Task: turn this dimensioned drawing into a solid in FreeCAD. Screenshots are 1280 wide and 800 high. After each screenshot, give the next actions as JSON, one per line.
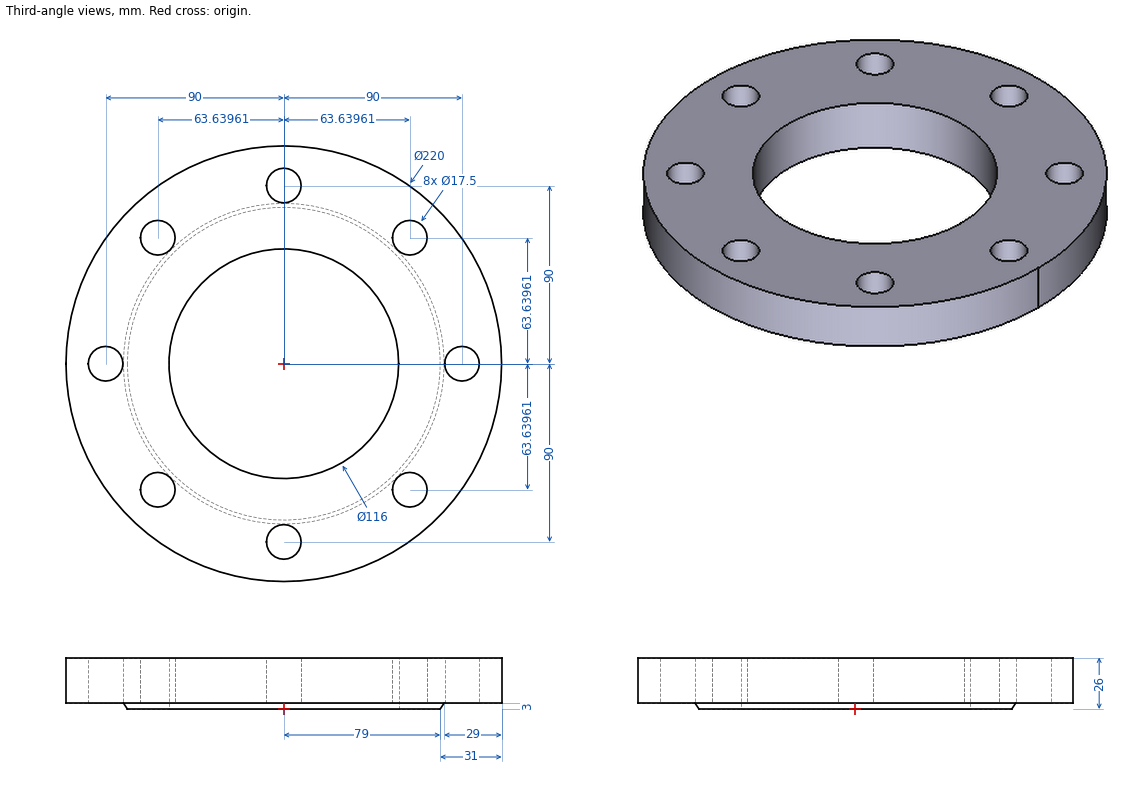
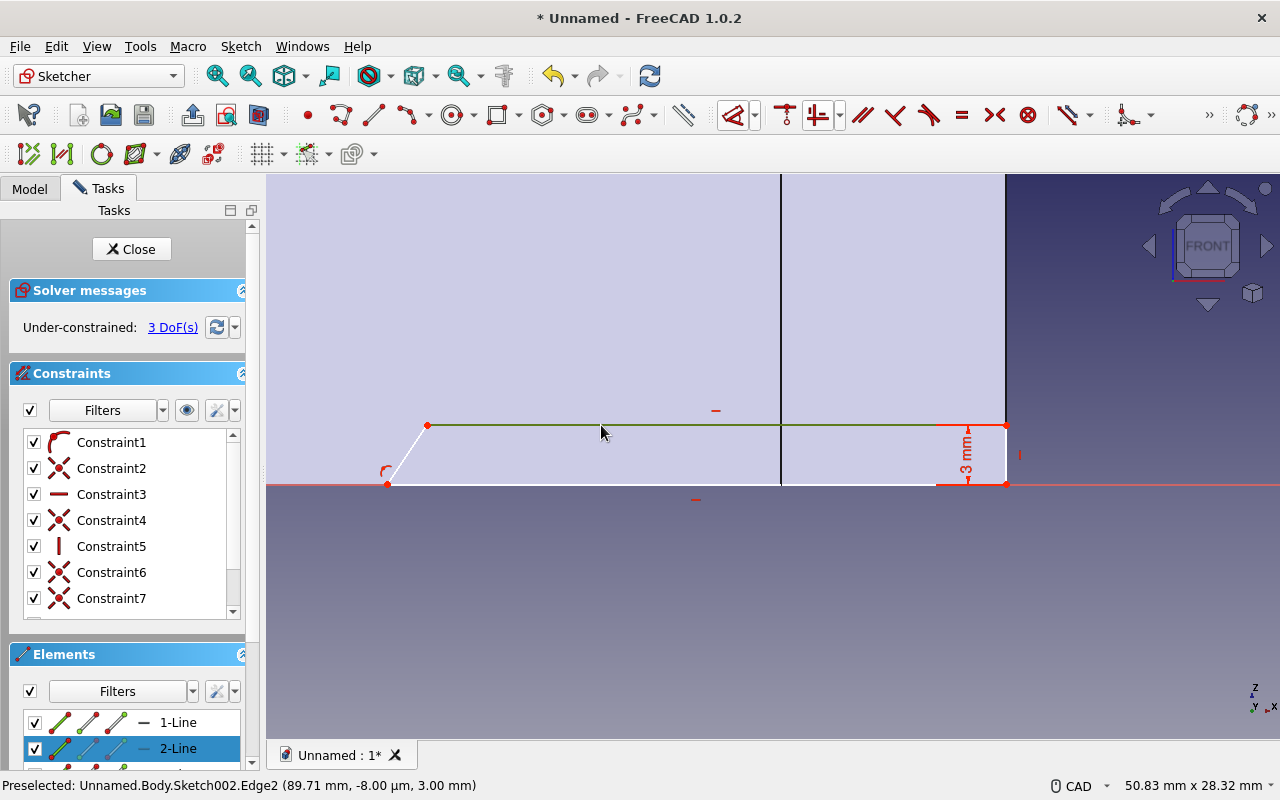
{"action": "key", "text": "l"}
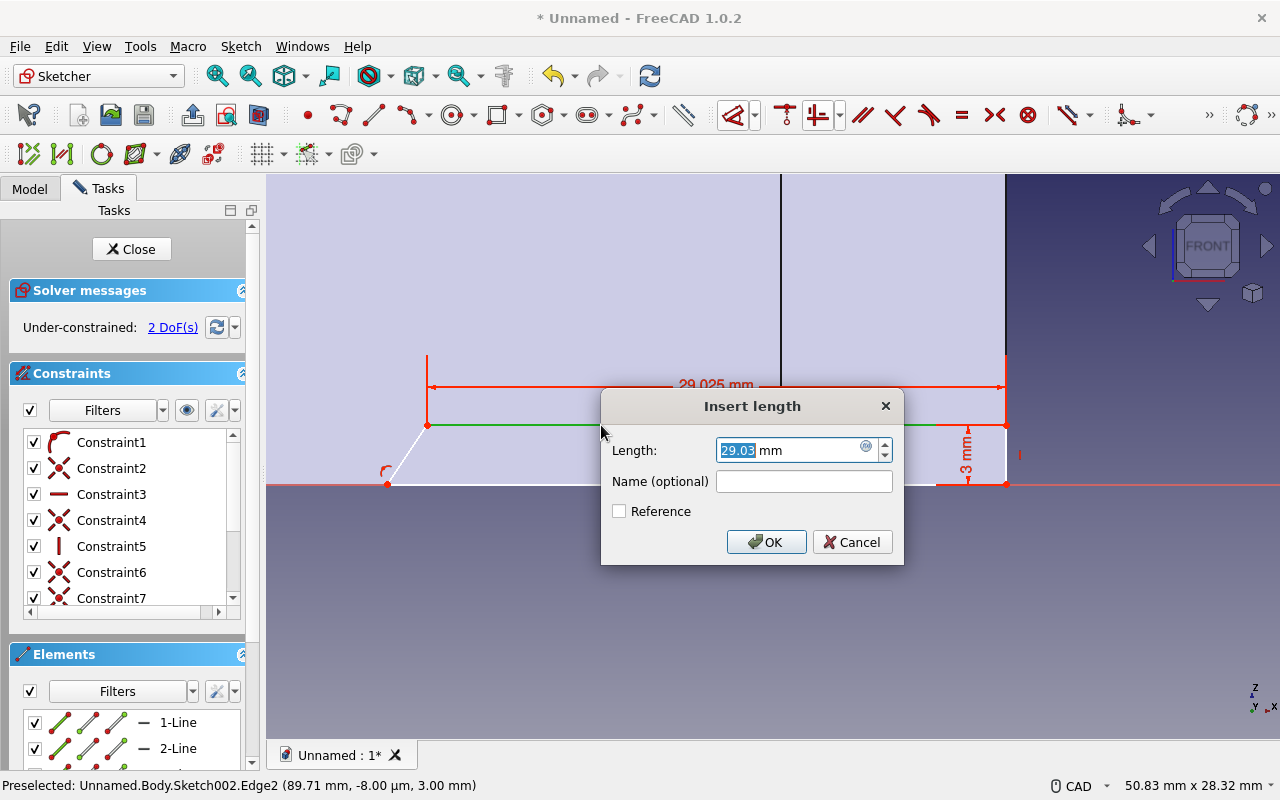
{"action": "type", "text": "29"}
{"action": "key", "text": "Return"}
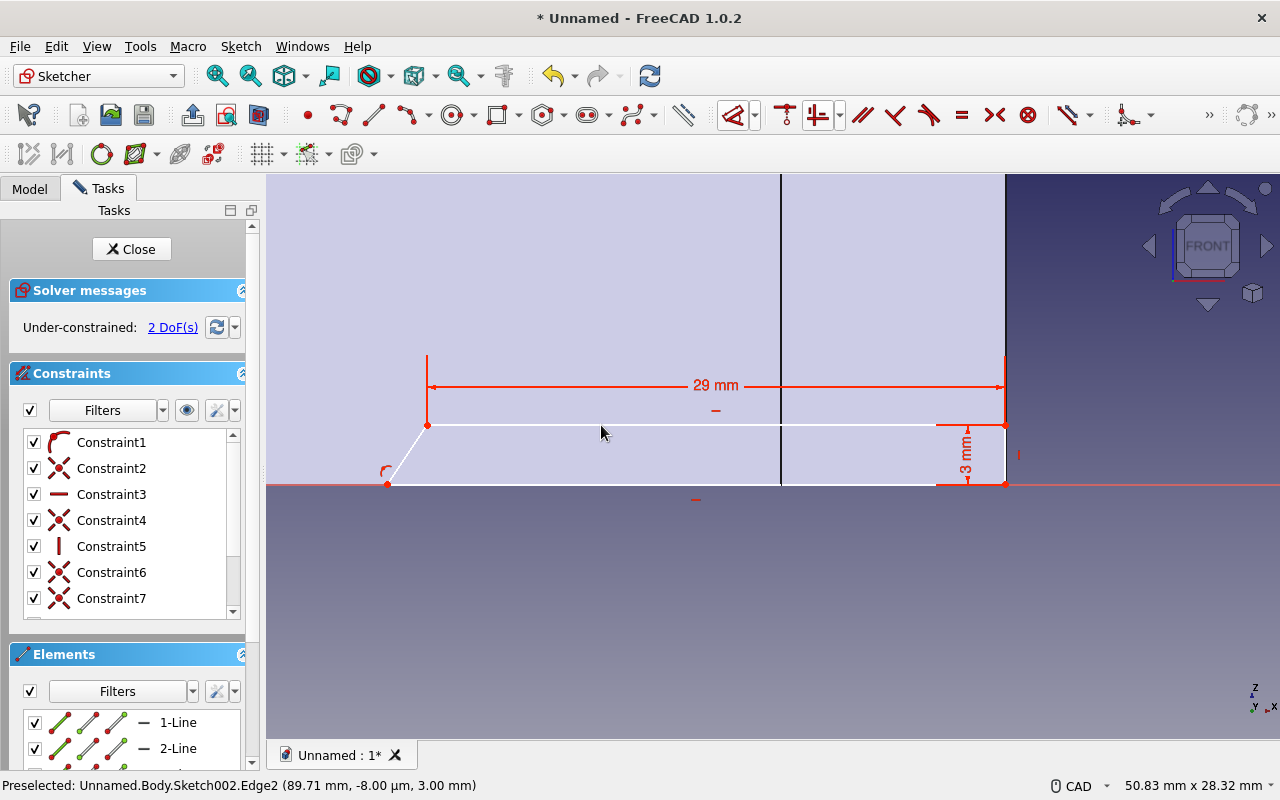
{"action": "left_click", "coordinate": [820, 485]}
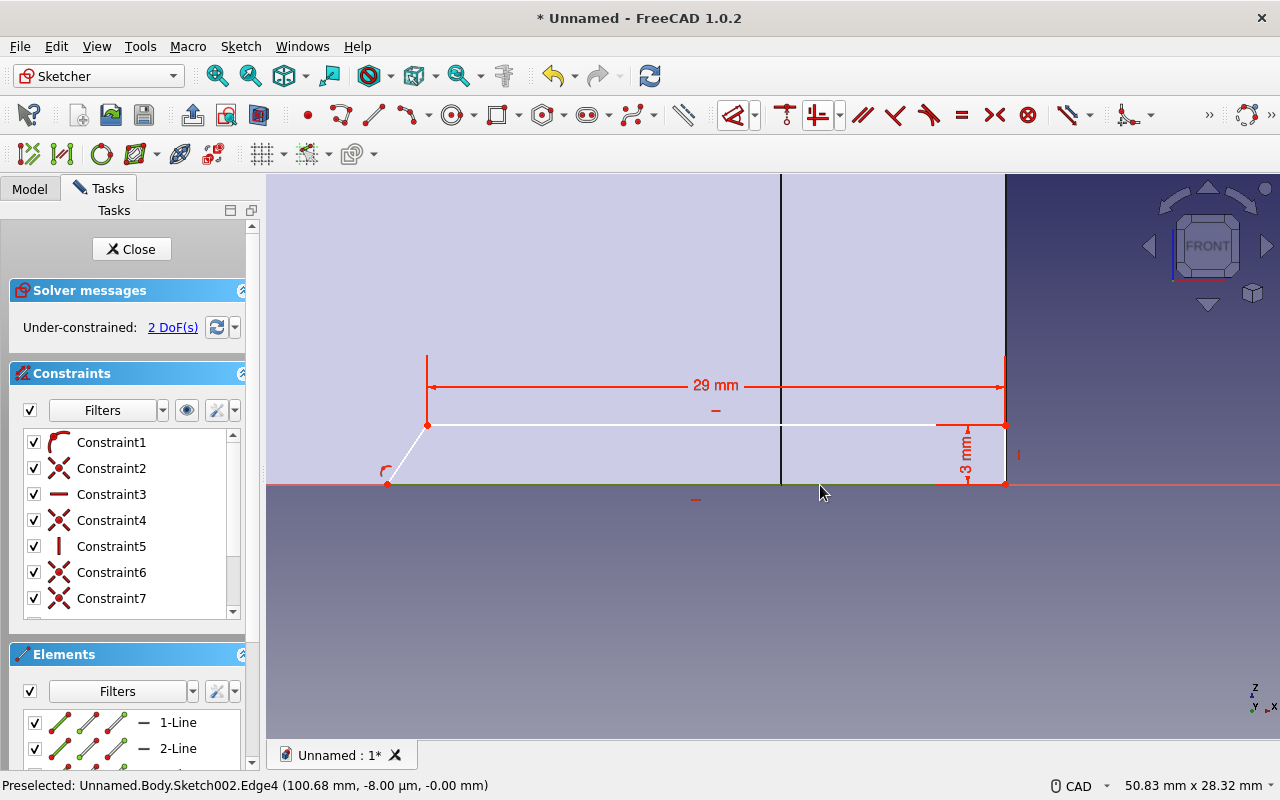
{"action": "key", "text": "l"}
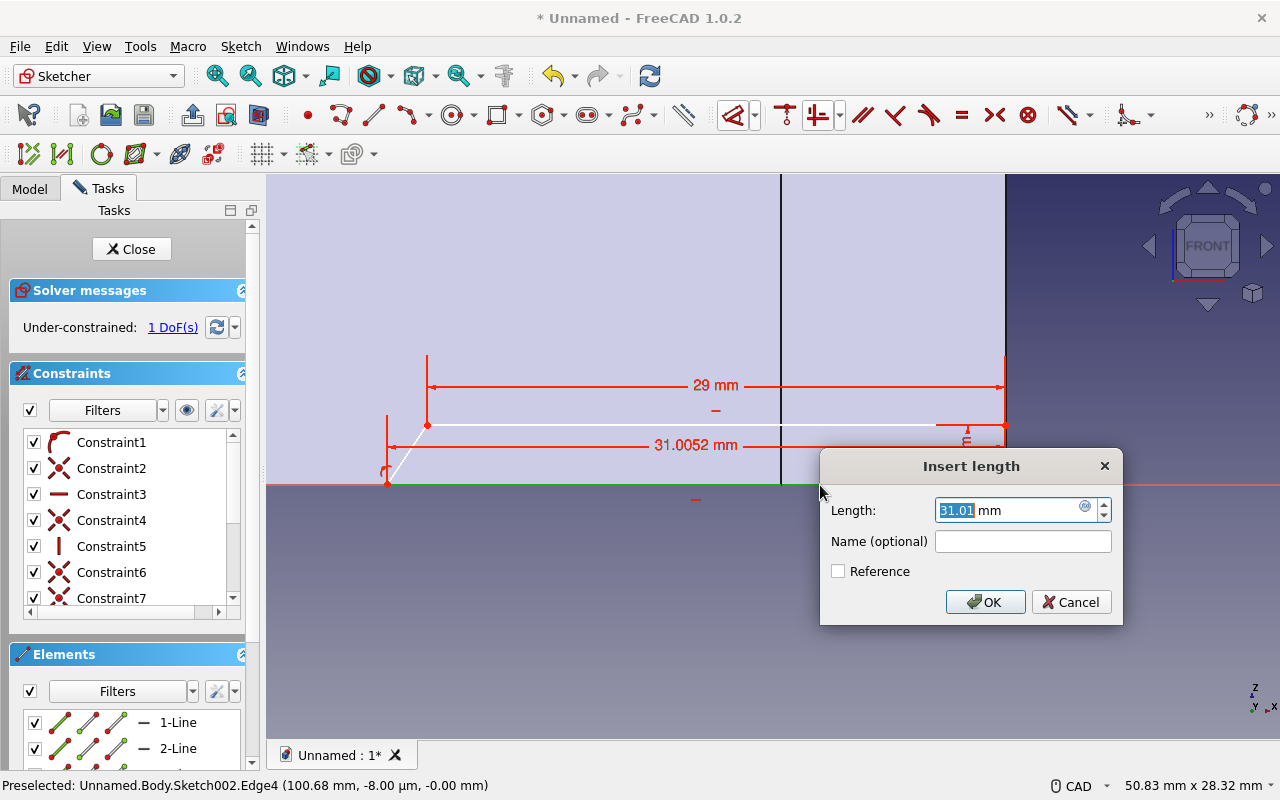
{"action": "type", "text": "31"}
{"action": "key", "text": "Return"}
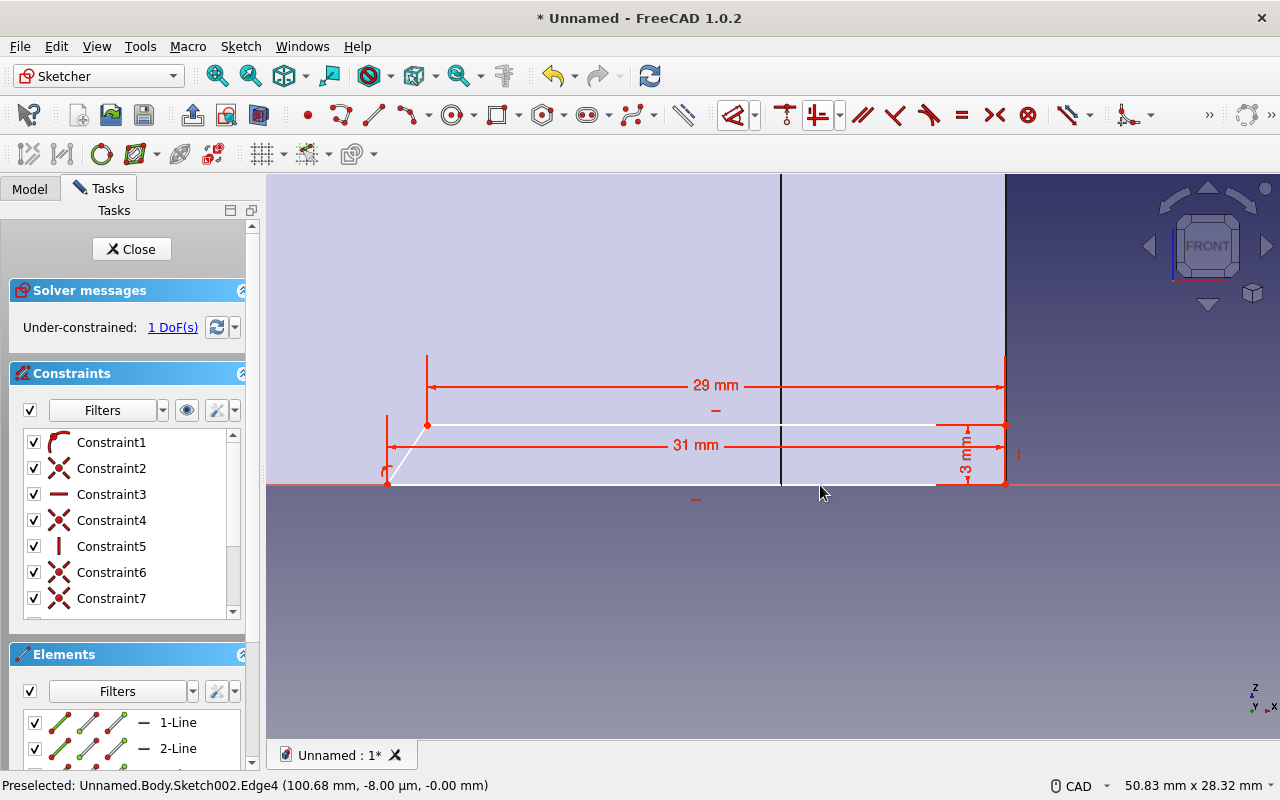
{"action": "left_click", "coordinate": [387, 485]}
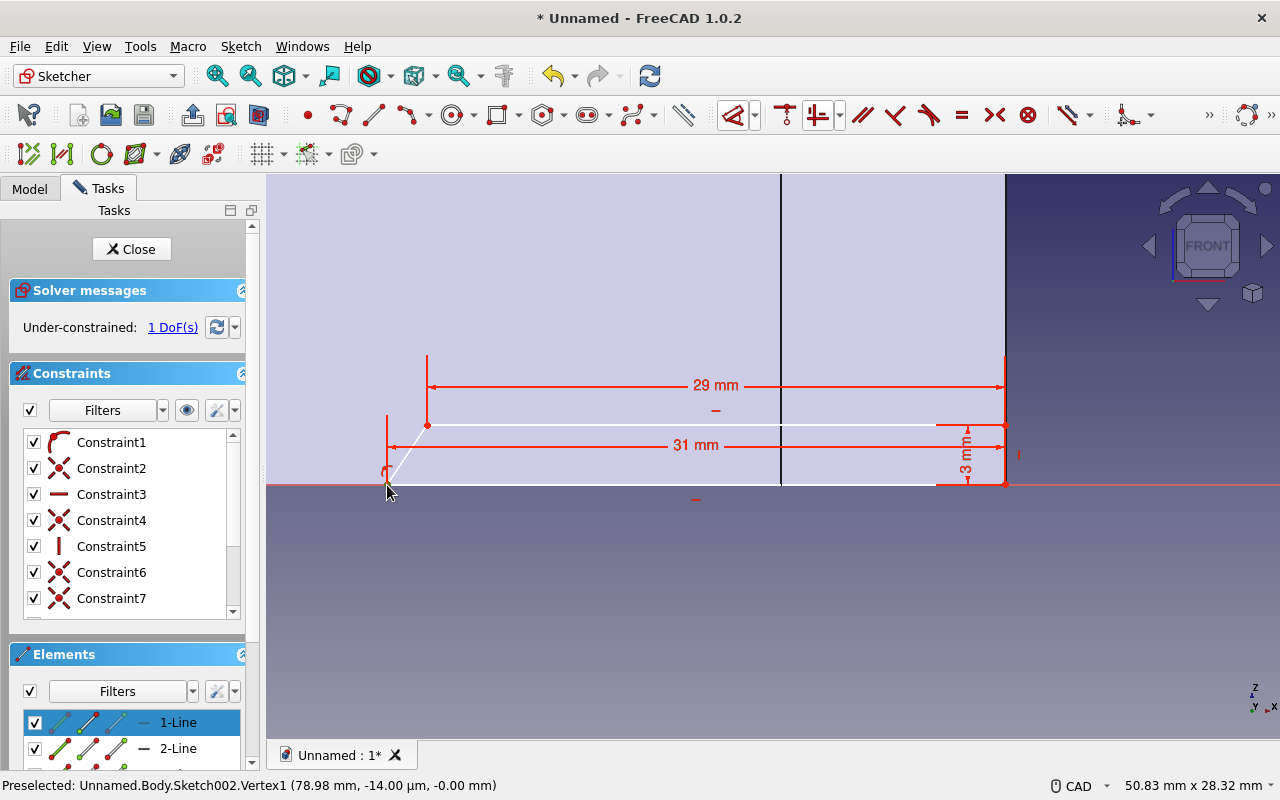
{"action": "left_click", "coordinate": [754, 116]}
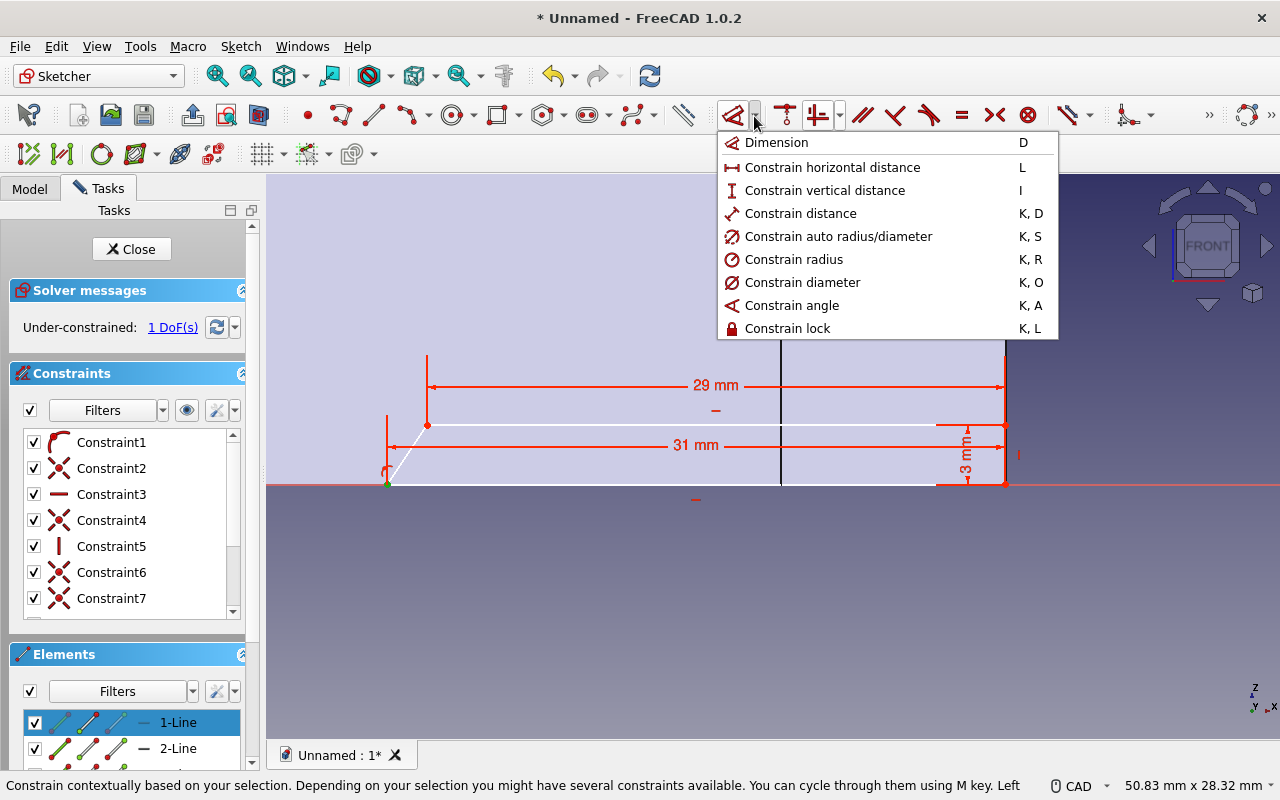
{"action": "left_click", "coordinate": [888, 168]}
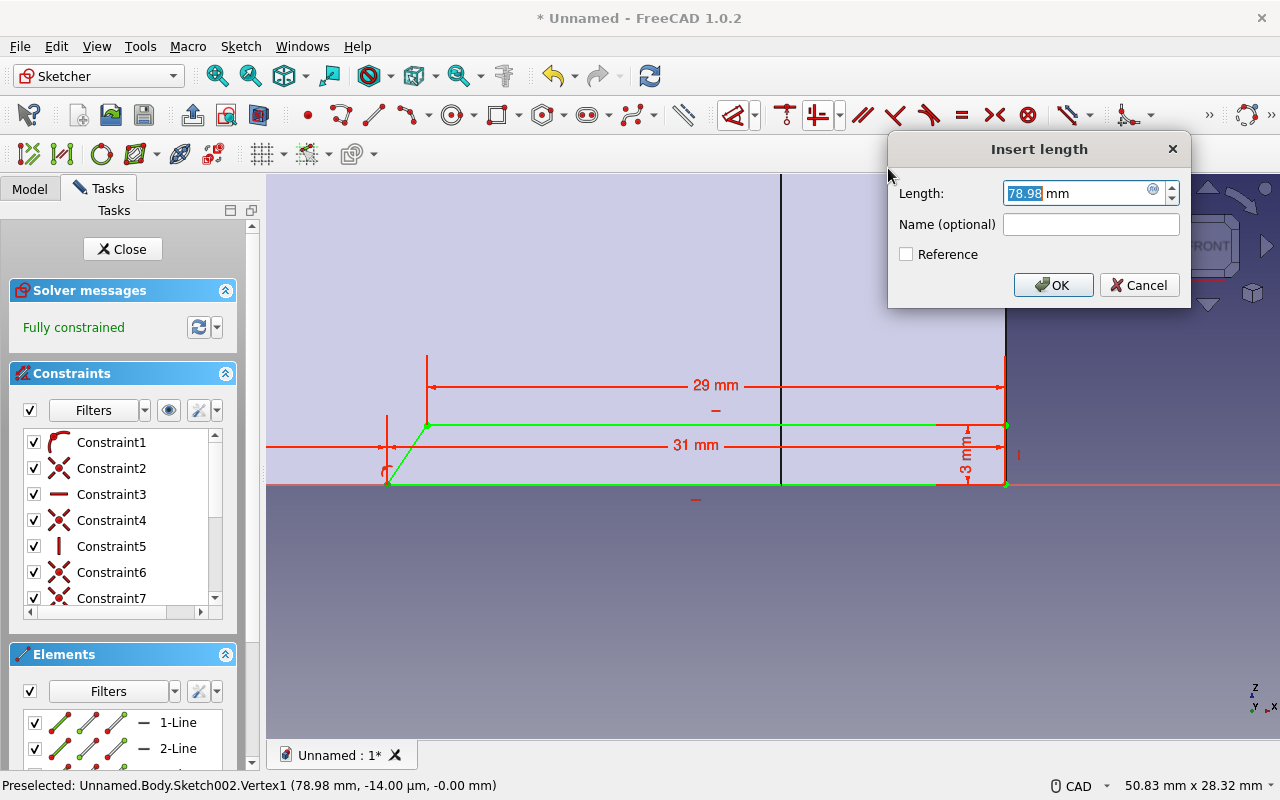
{"action": "type", "text": "79"}
{"action": "key", "text": "Return"}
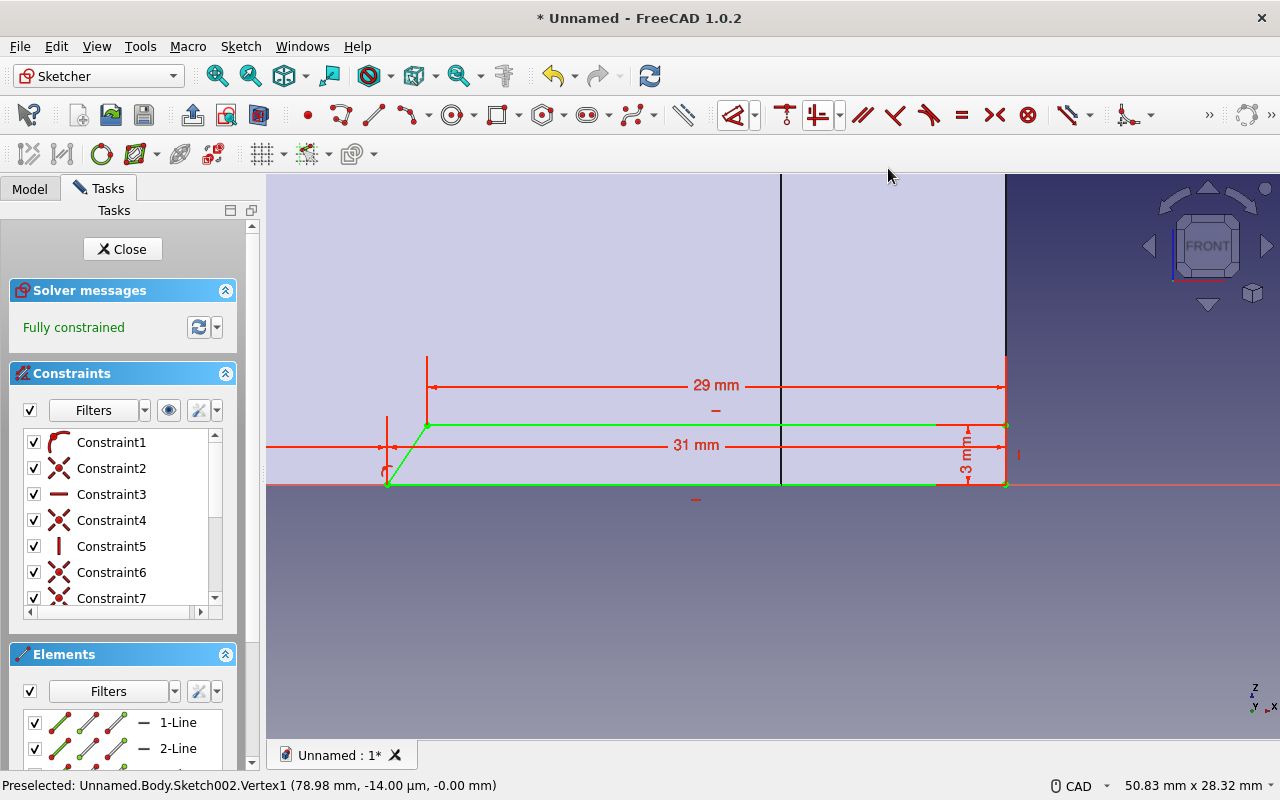
{"action": "left_click", "coordinate": [123, 249]}